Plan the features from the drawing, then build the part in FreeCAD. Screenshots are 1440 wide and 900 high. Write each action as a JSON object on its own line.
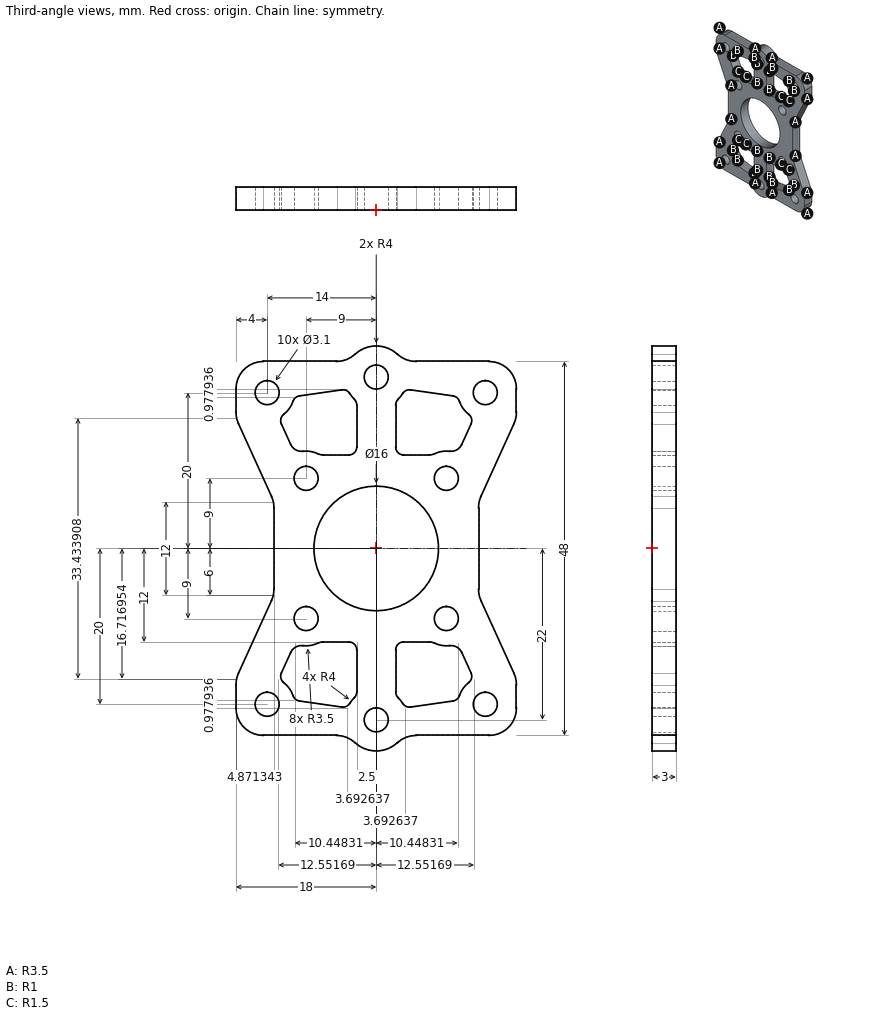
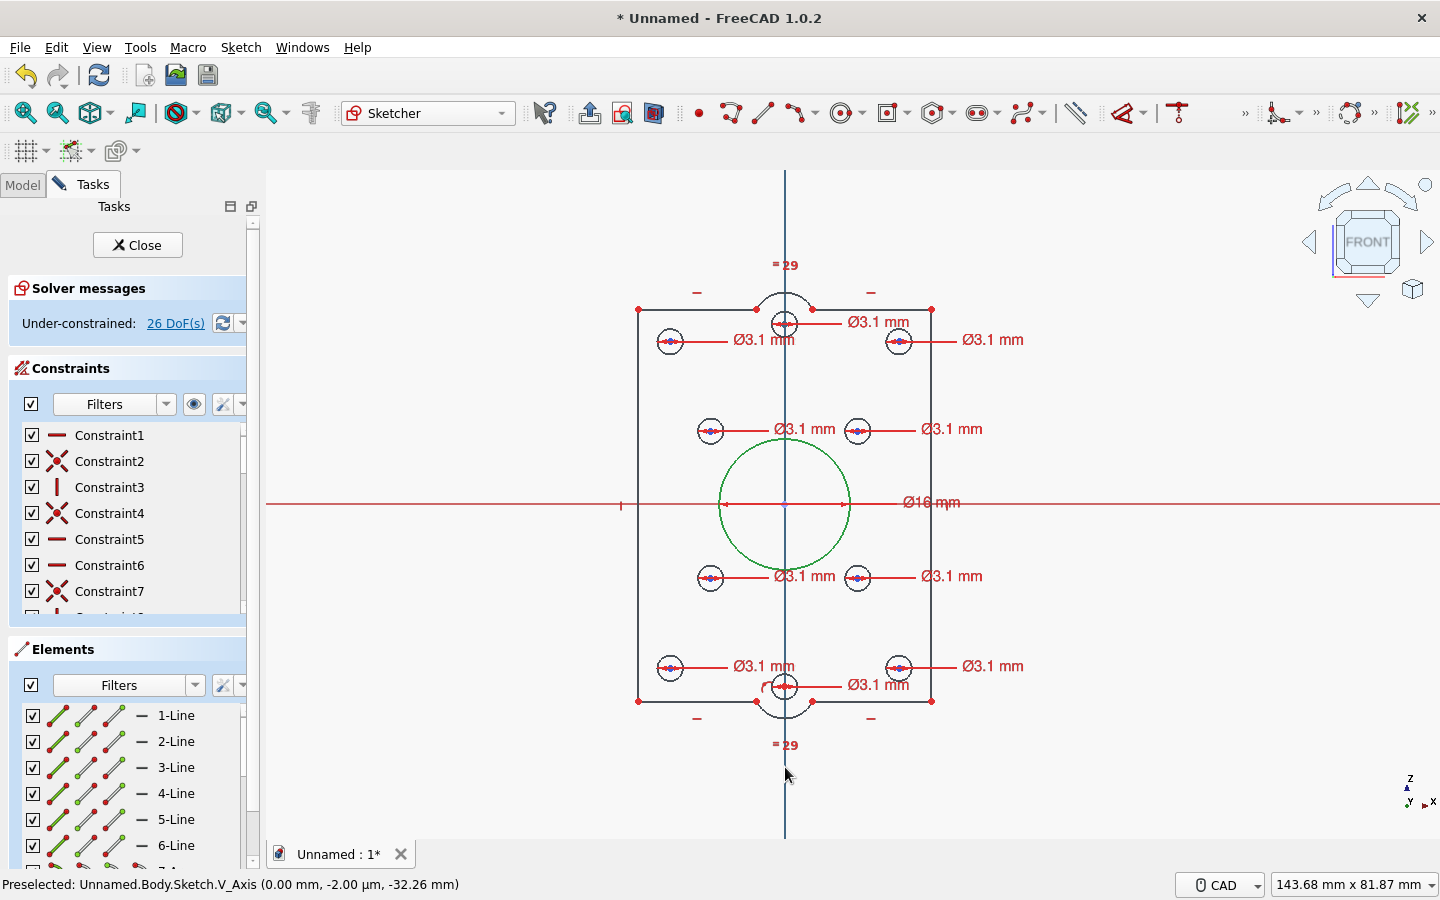
{"action": "left_click", "coordinate": [1178, 114]}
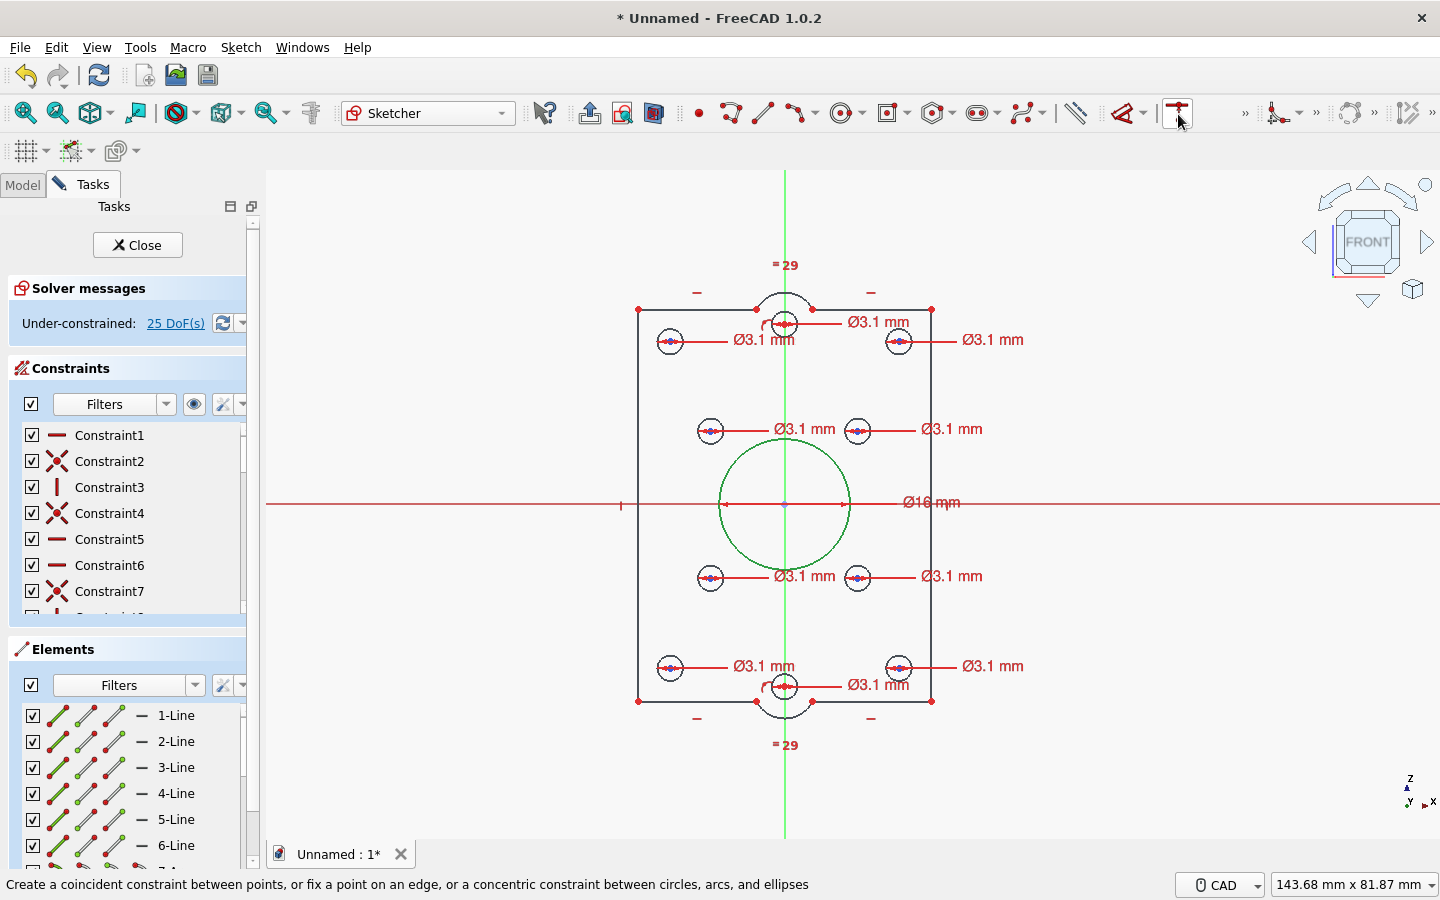
{"action": "left_click", "coordinate": [711, 431]}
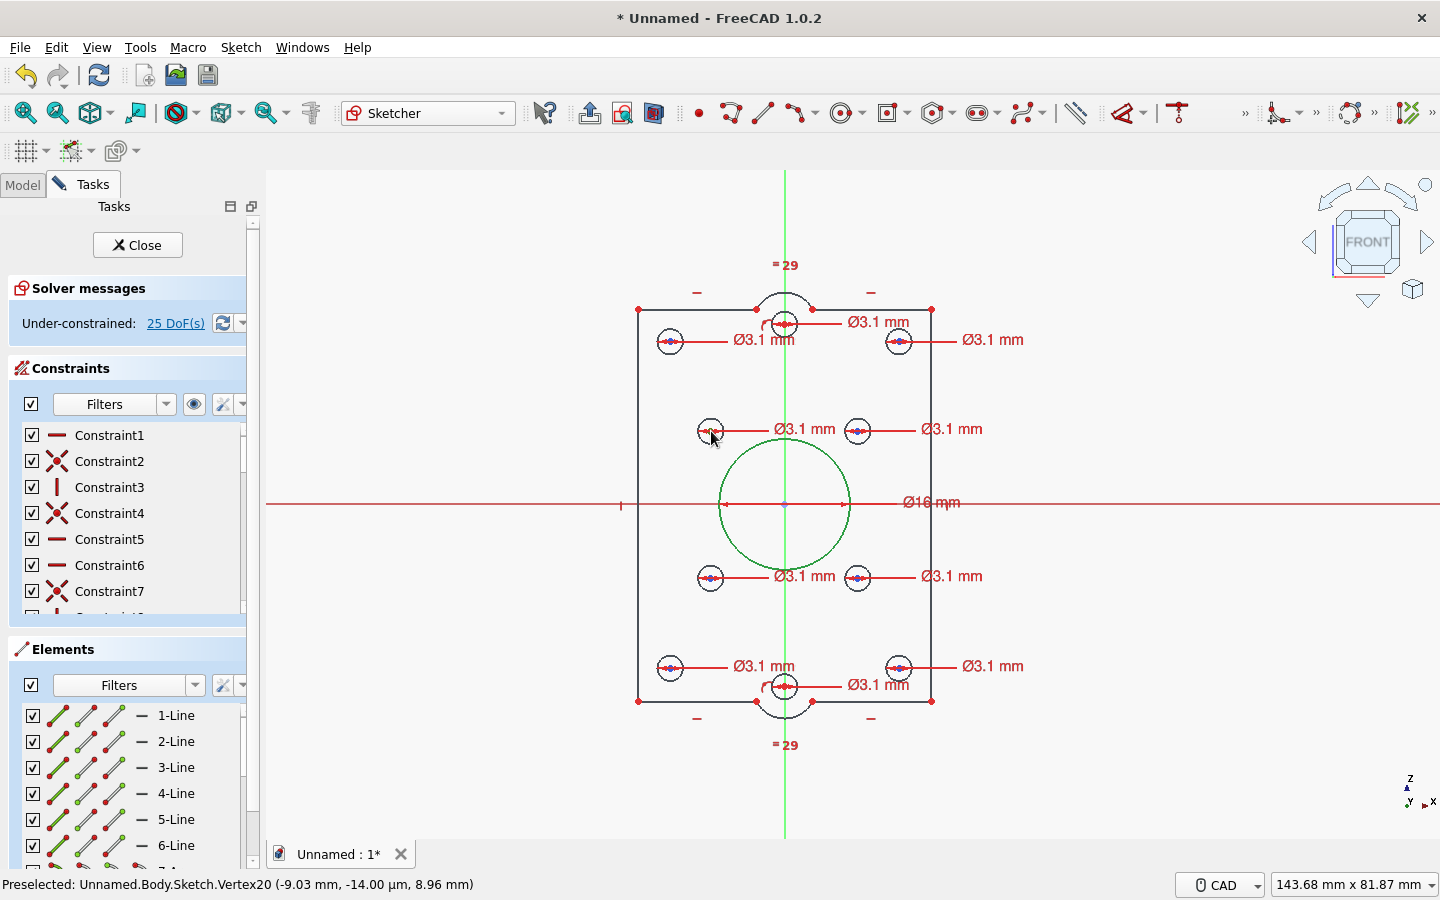
{"action": "left_click", "coordinate": [858, 431]}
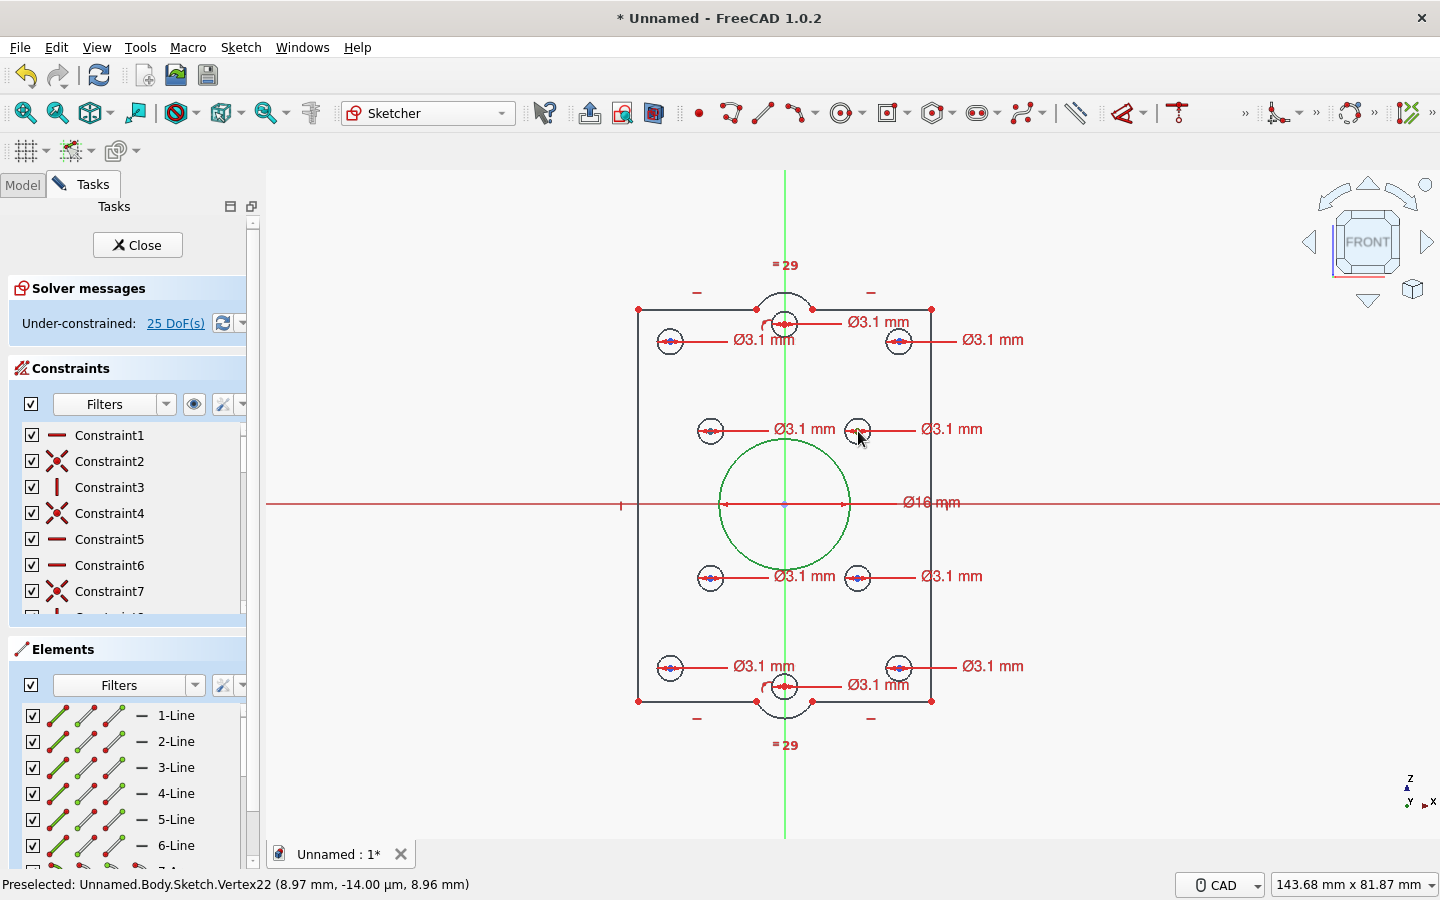
{"action": "key", "text": "h"}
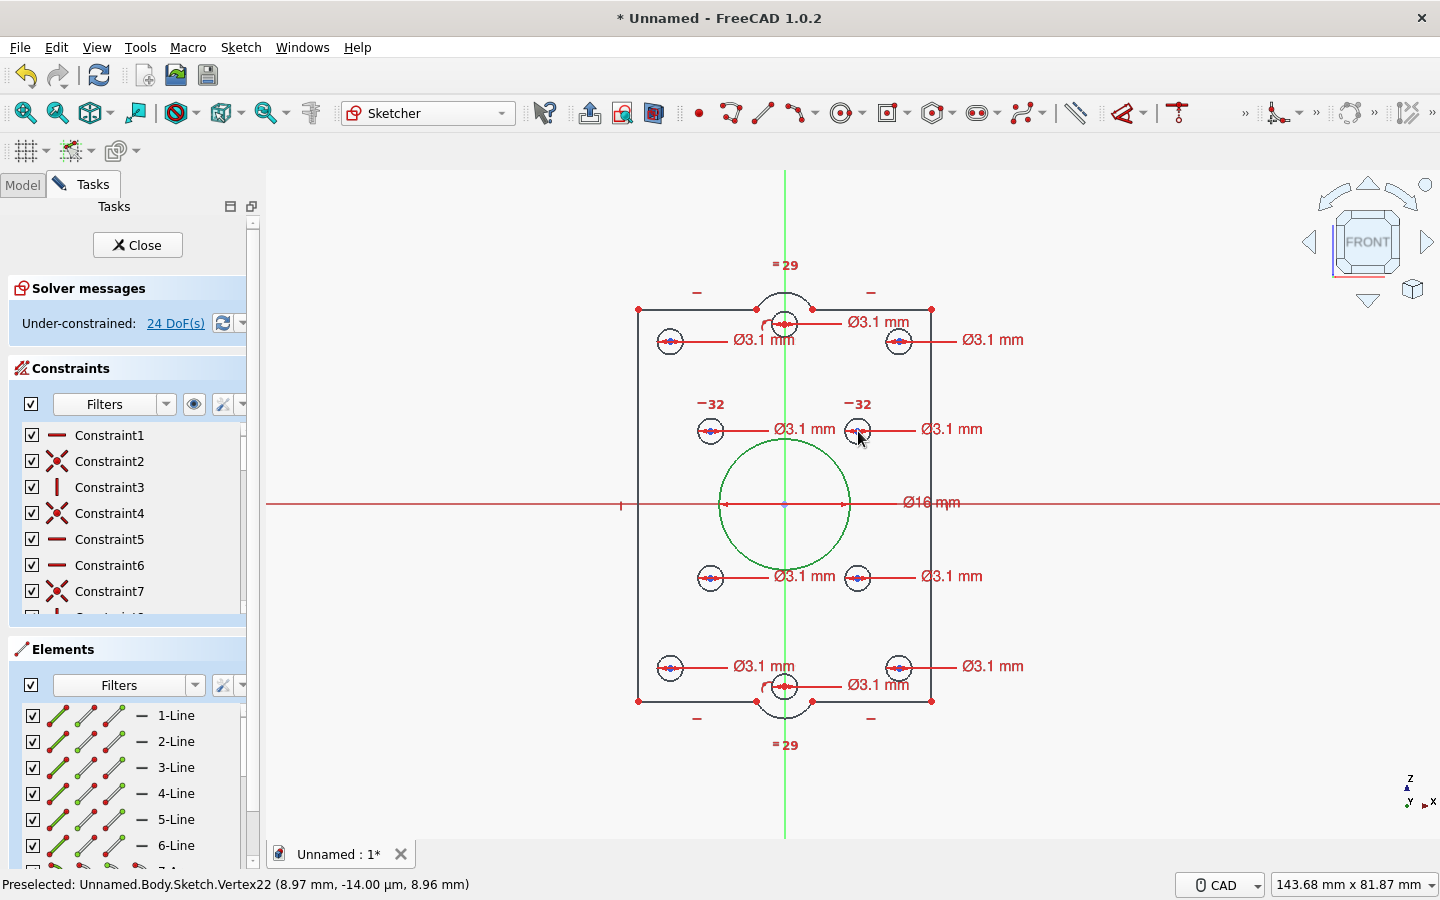
{"action": "left_click", "coordinate": [711, 431]}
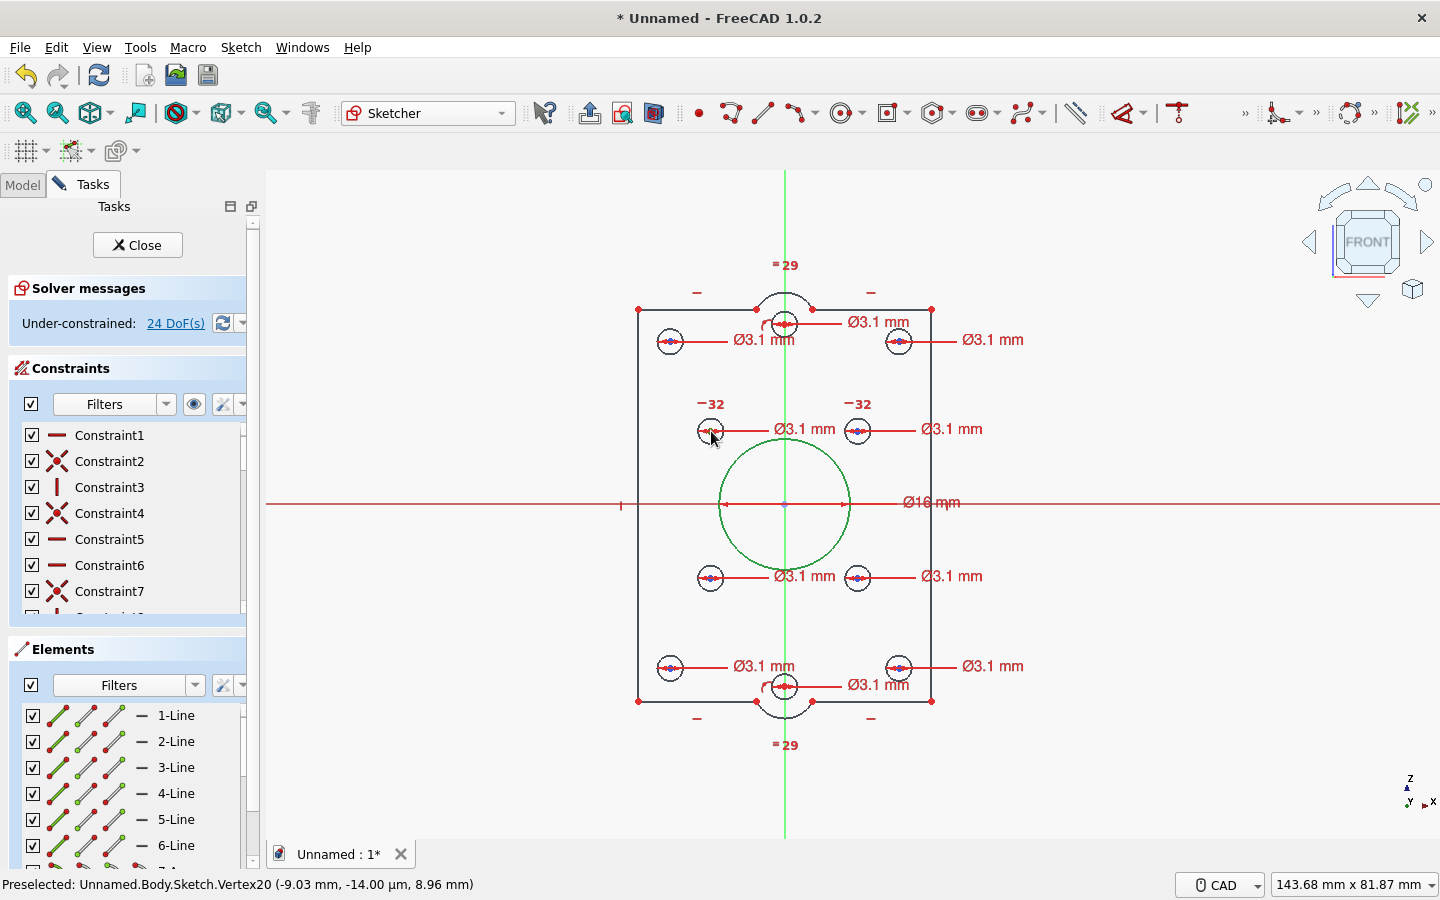
{"action": "left_click", "coordinate": [711, 578]}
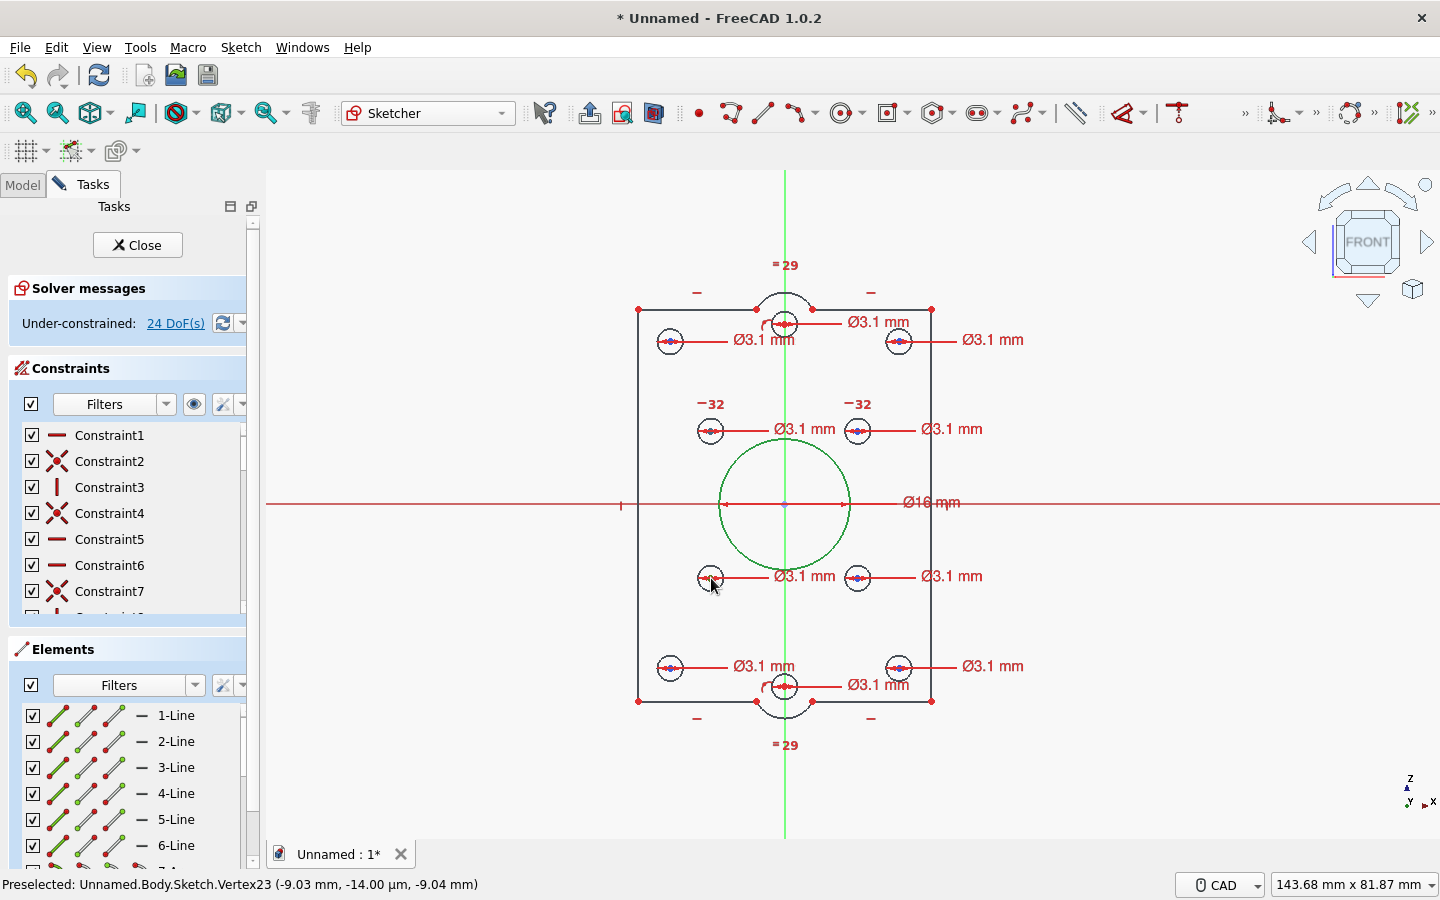
{"action": "key", "text": "v"}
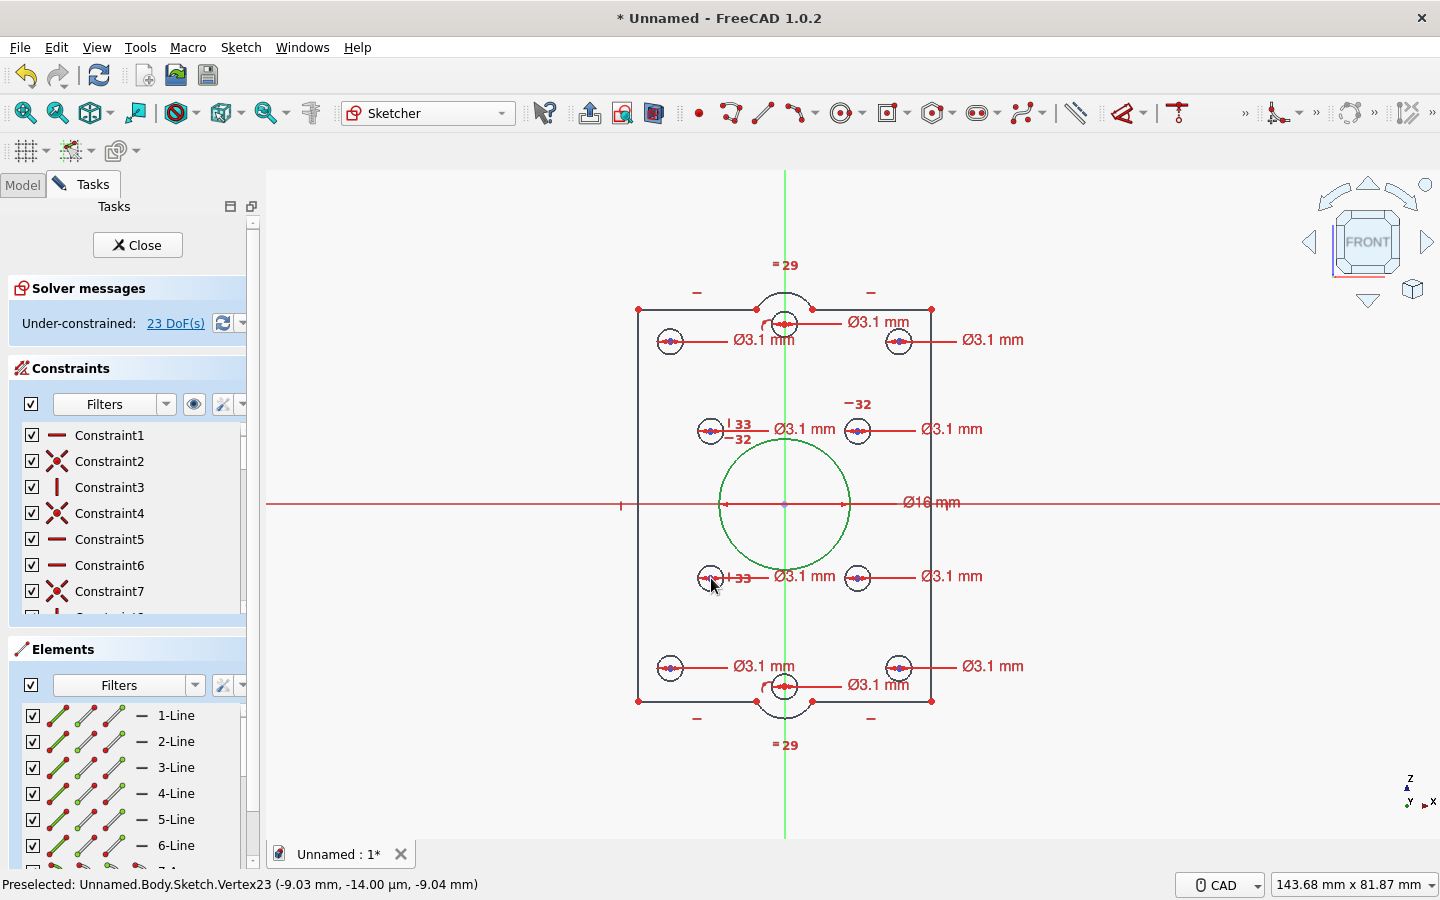
{"action": "left_click", "coordinate": [858, 431]}